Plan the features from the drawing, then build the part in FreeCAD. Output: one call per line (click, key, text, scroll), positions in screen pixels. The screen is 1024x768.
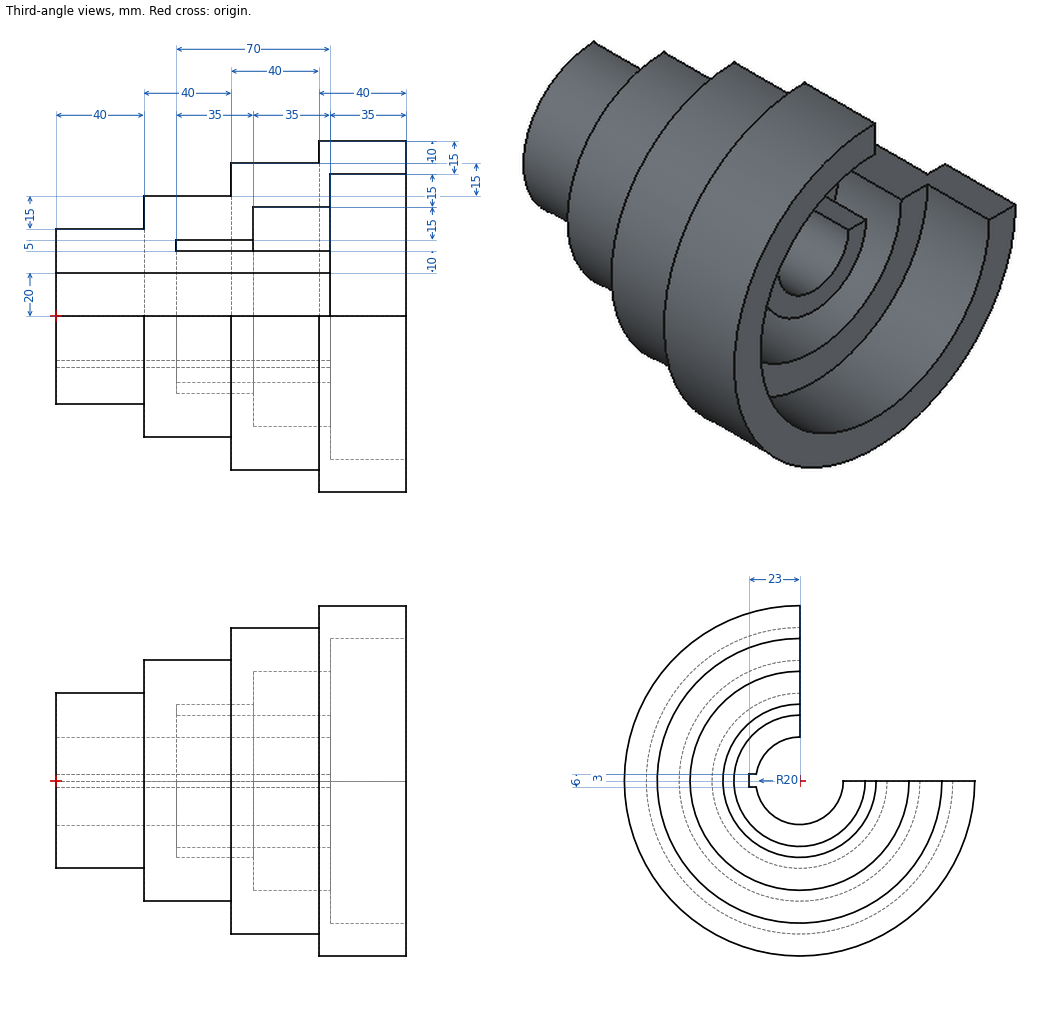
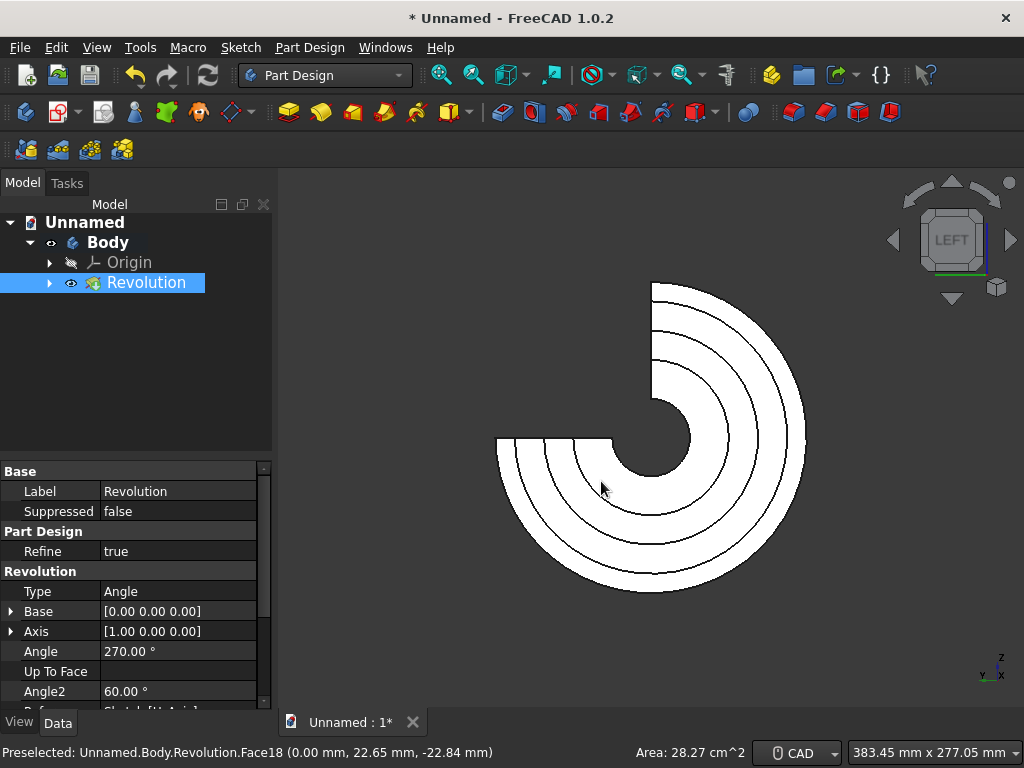
click(58, 112)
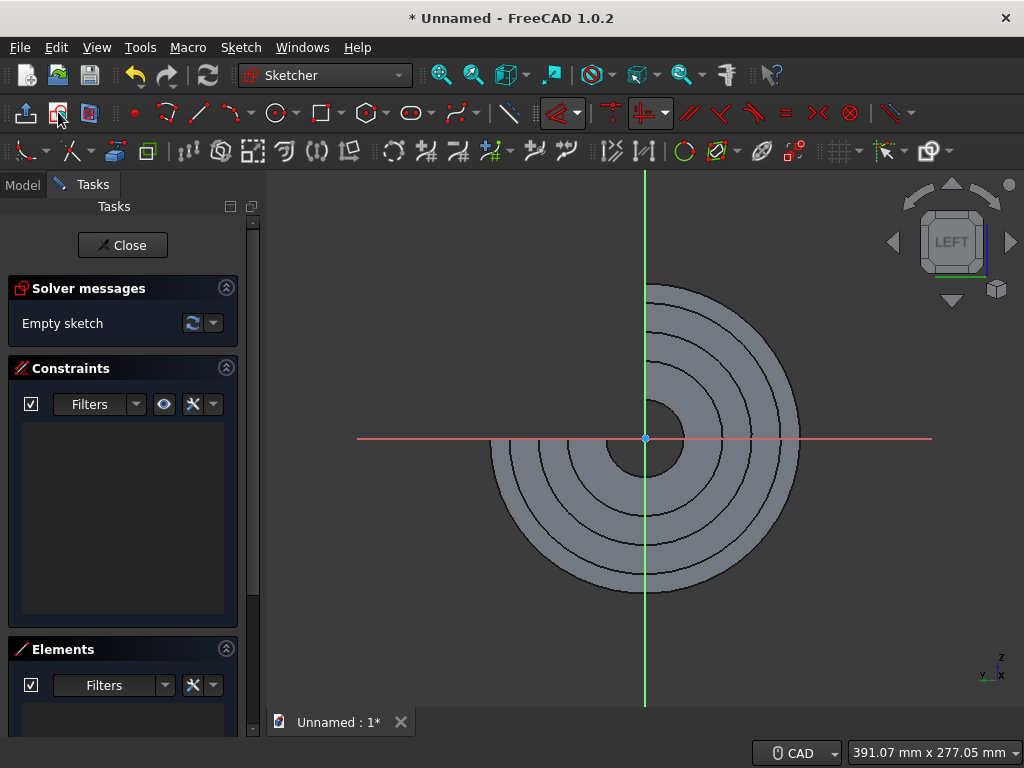
scroll(692, 439, up, 15)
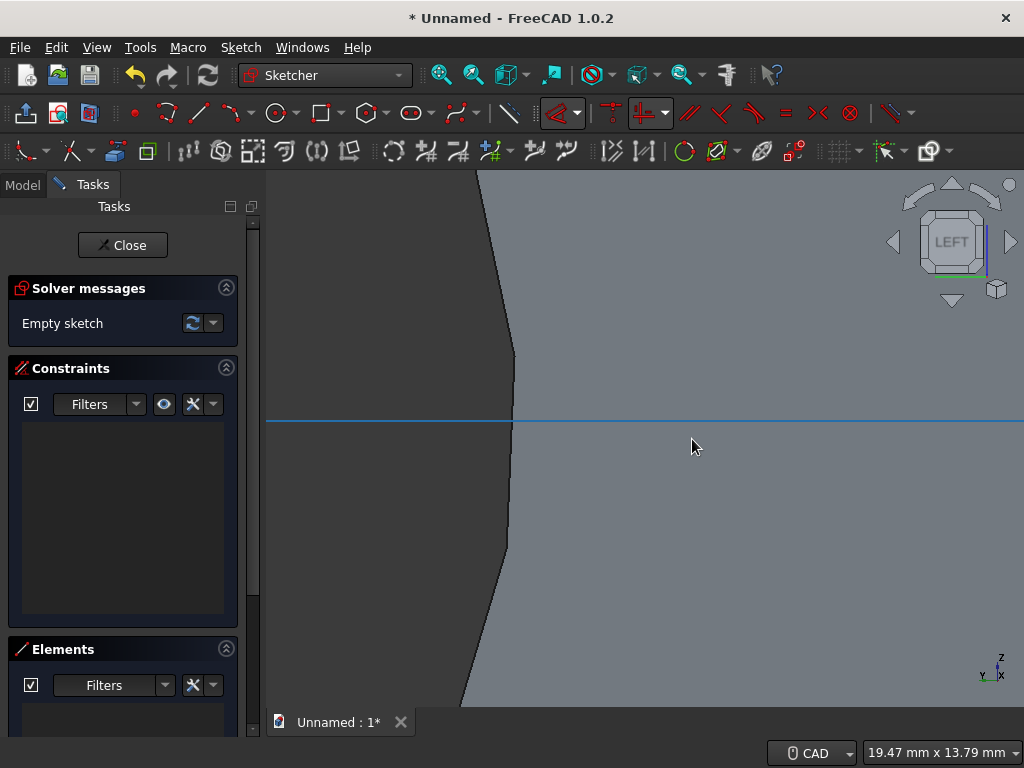
scroll(560, 385, up, 2)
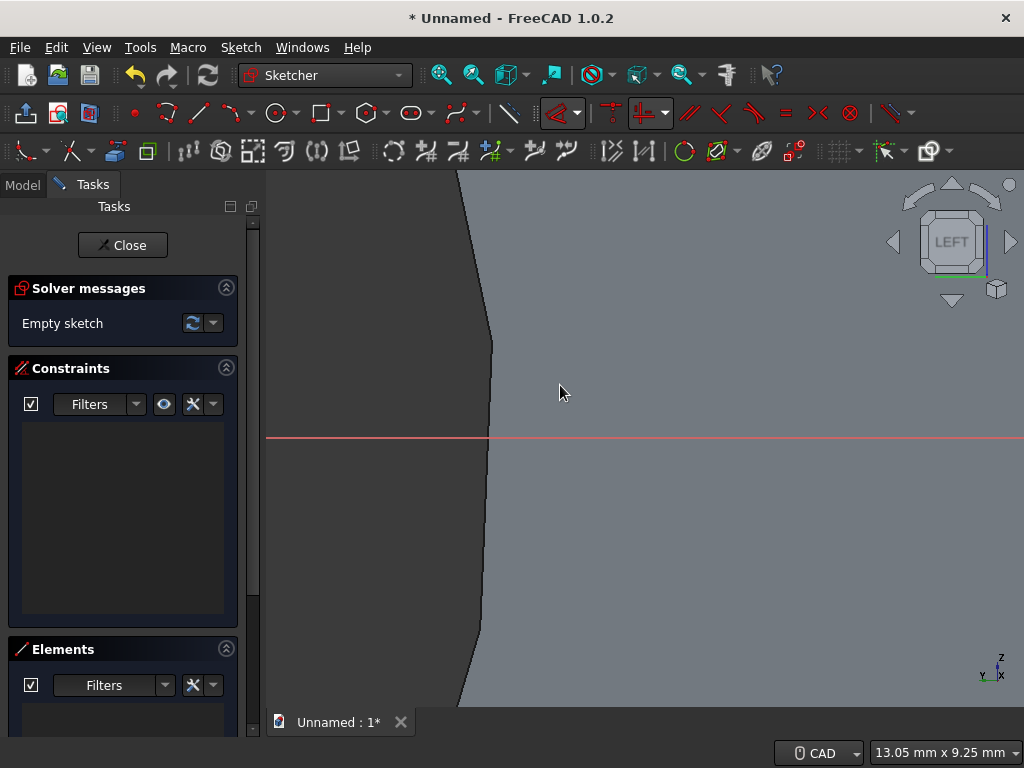
click(168, 114)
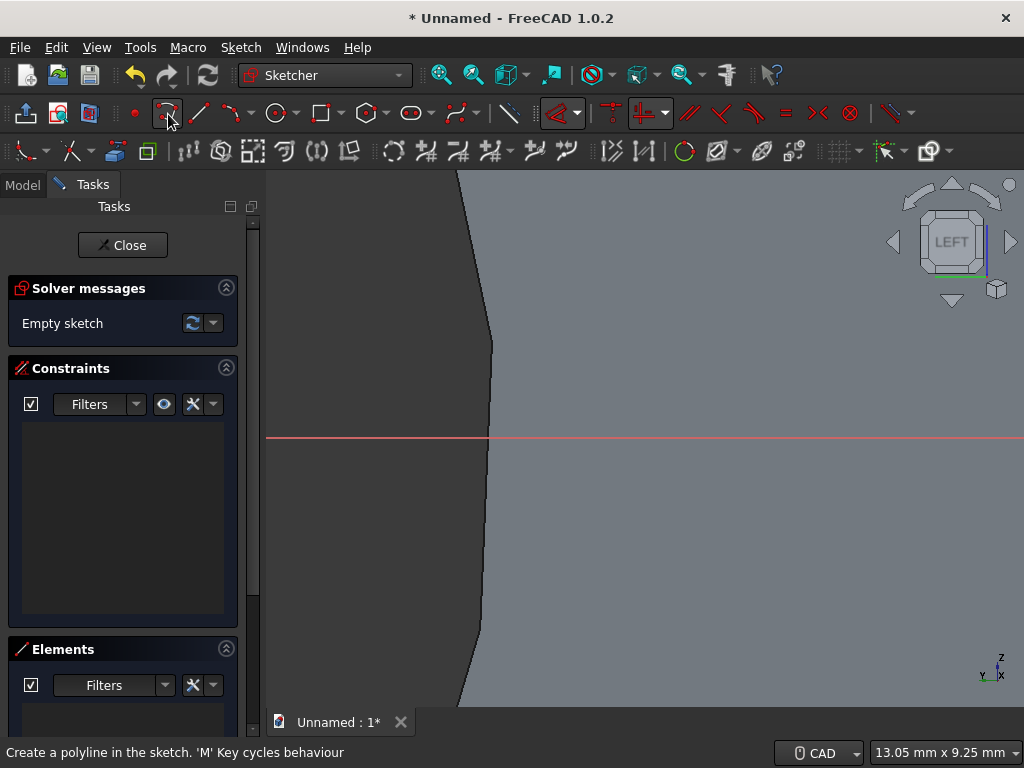
click(483, 264)
click(670, 264)
click(670, 612)
click(483, 612)
right_click(483, 612)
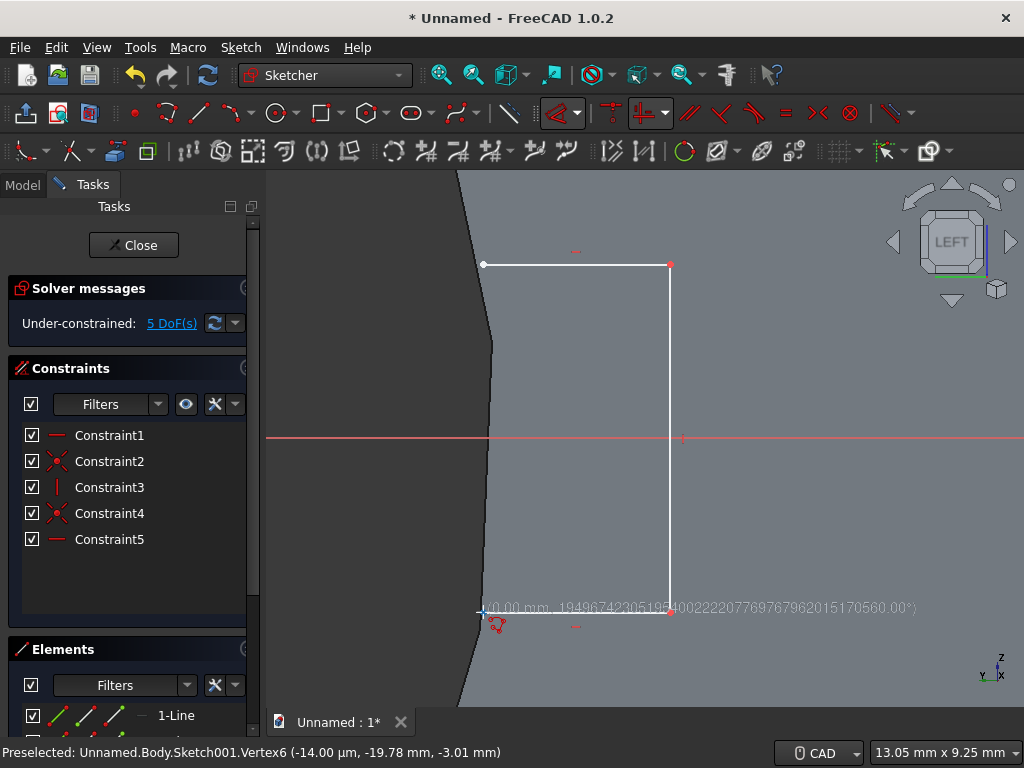
click(232, 114)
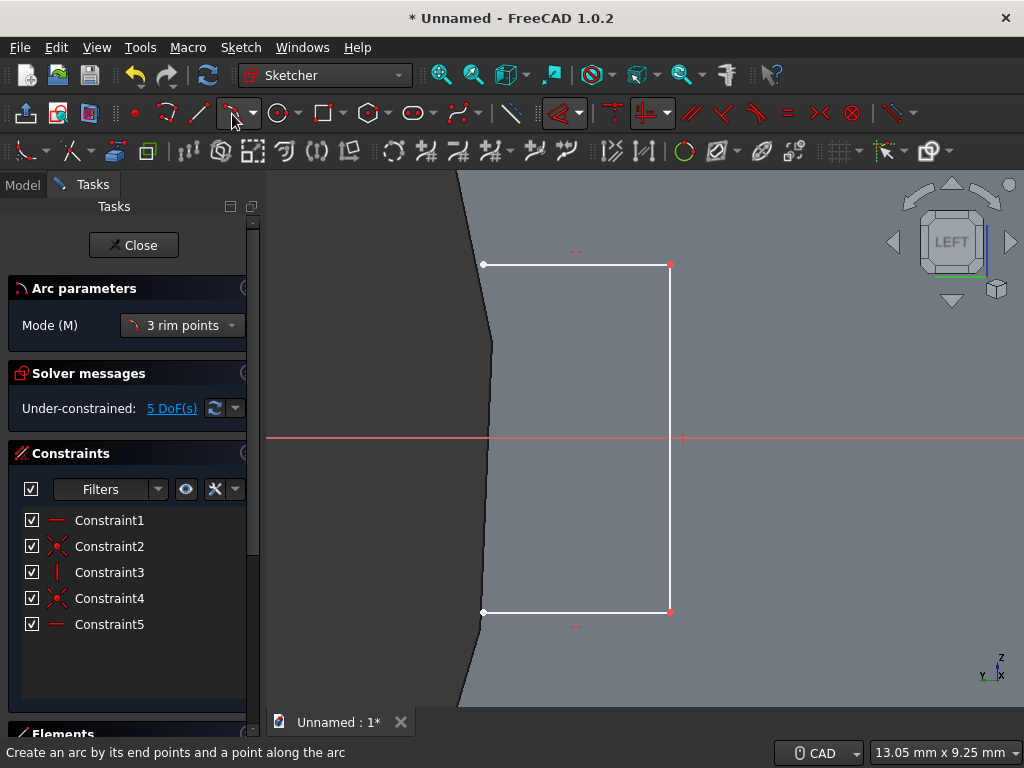
click(483, 613)
click(483, 265)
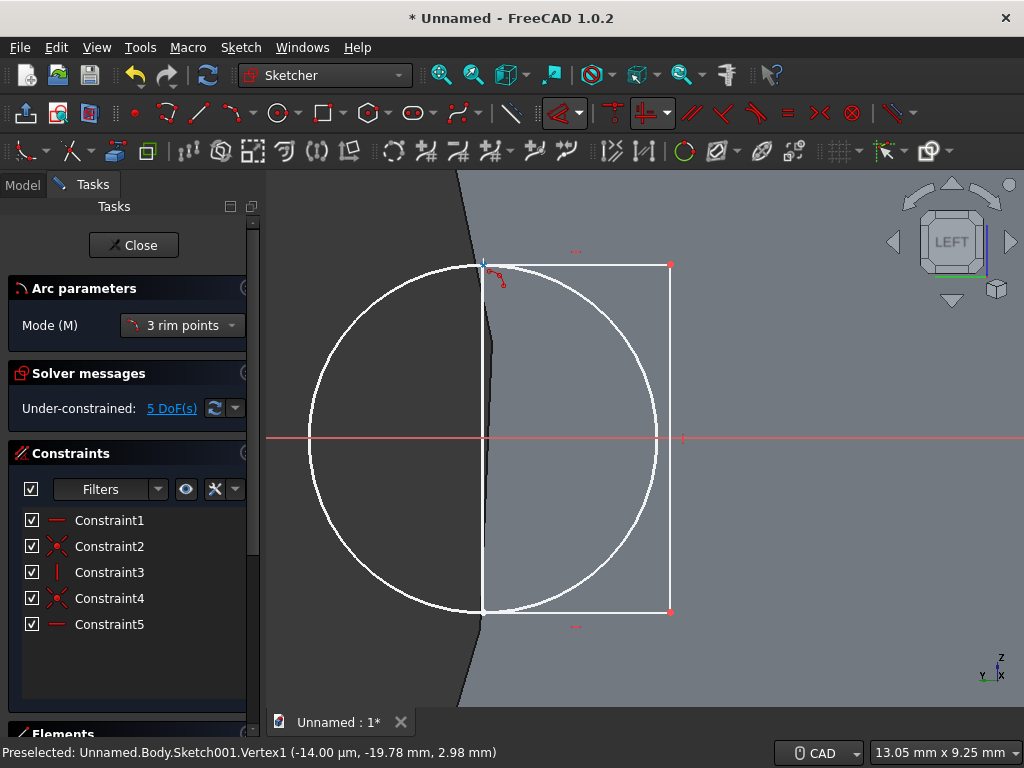
scroll(495, 473, up, 2)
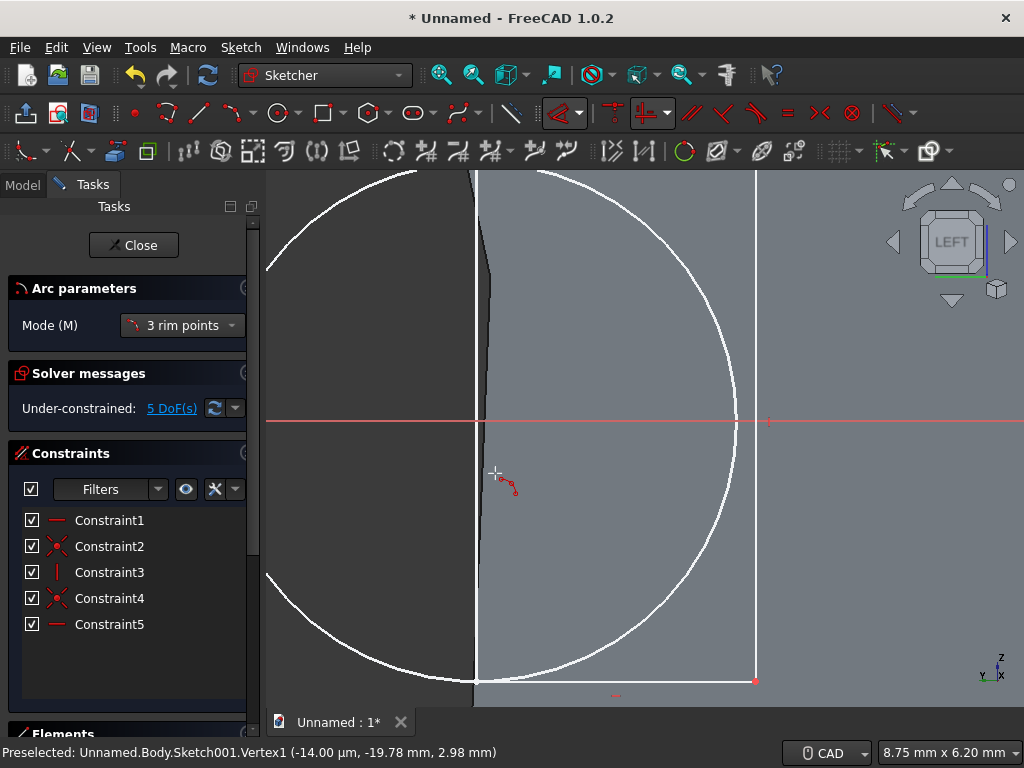
click(495, 473)
key(Escape)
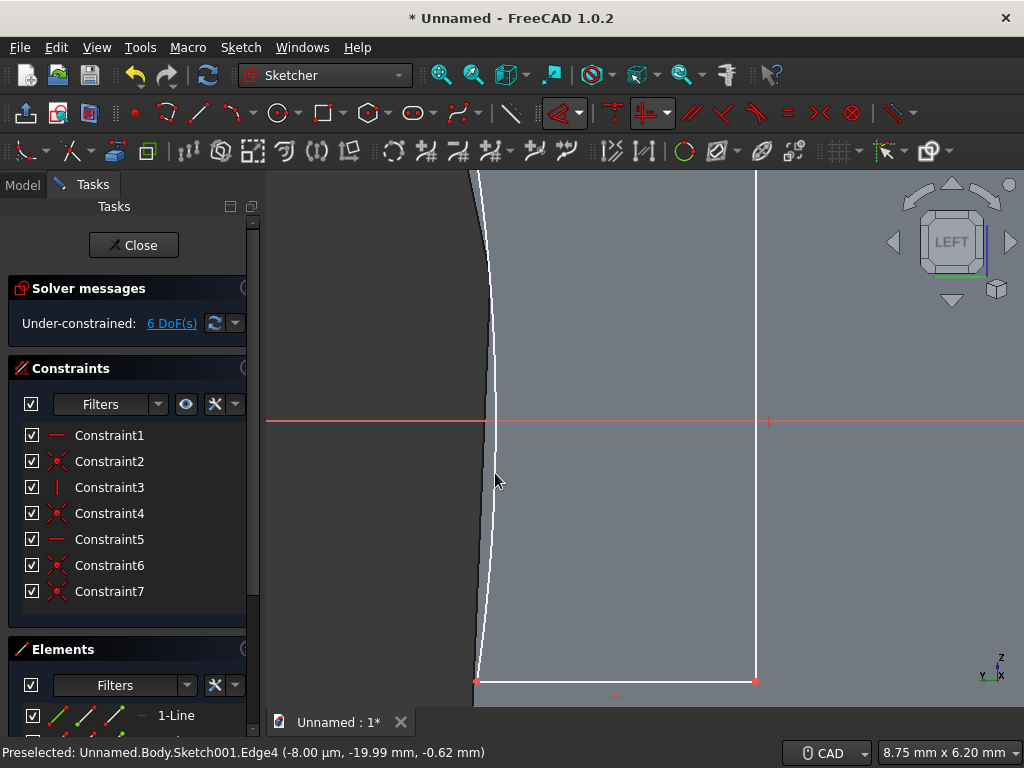
scroll(495, 475, down, 2)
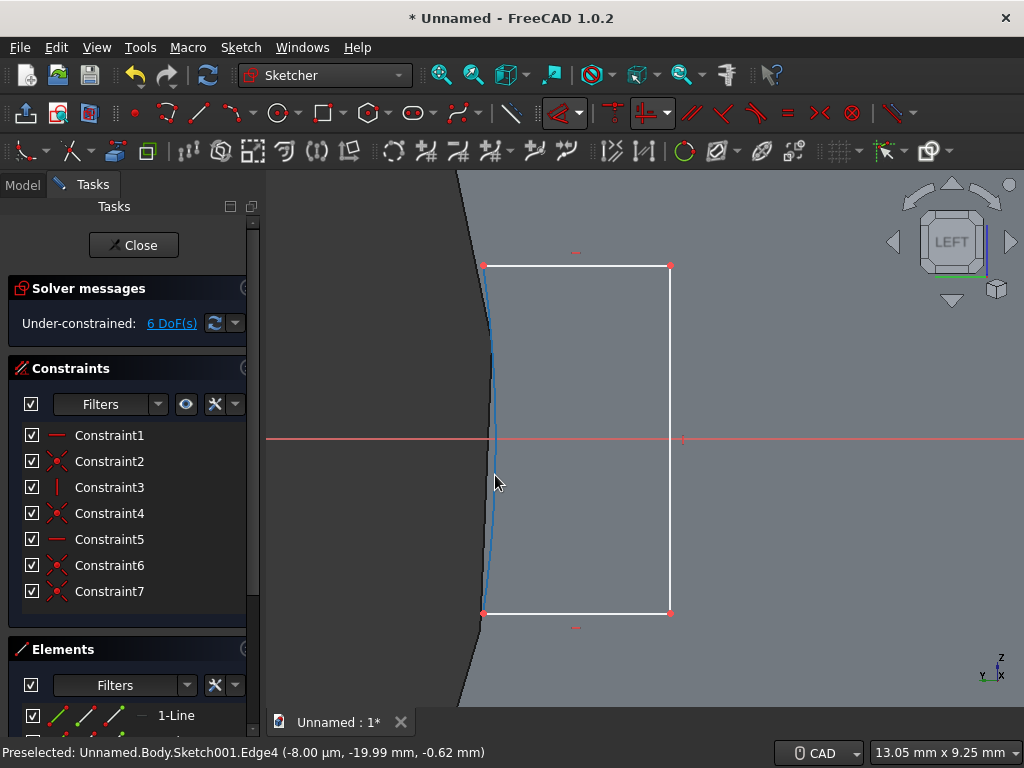
scroll(829, 438, down, 6)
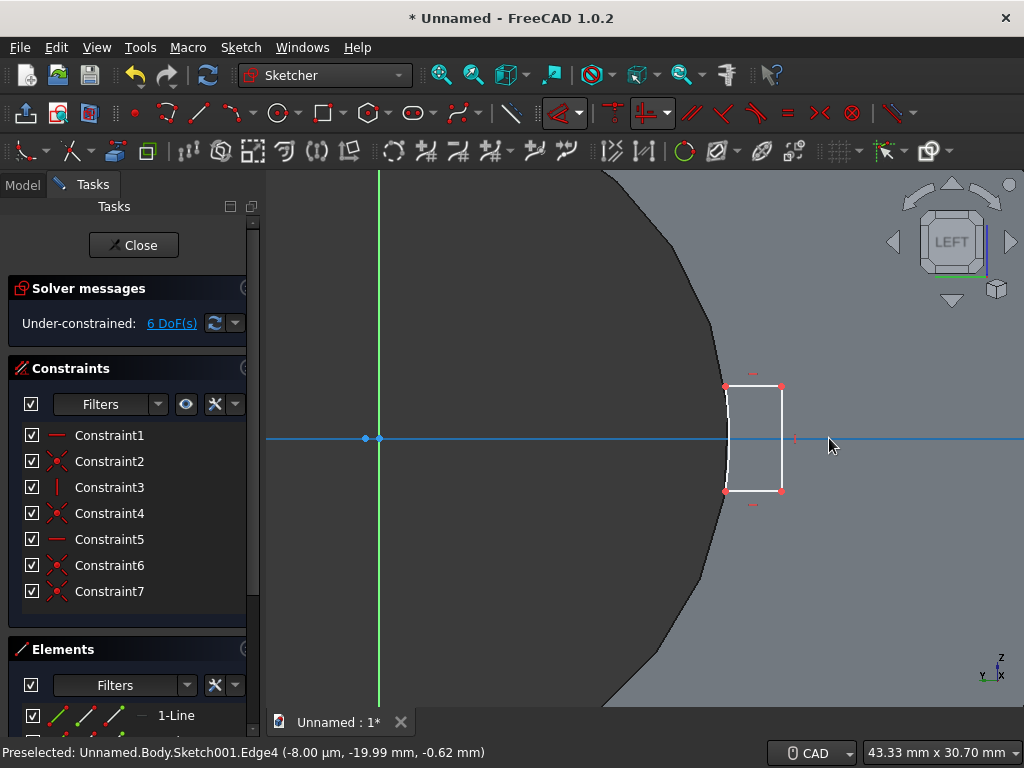
drag(355, 429, 389, 449)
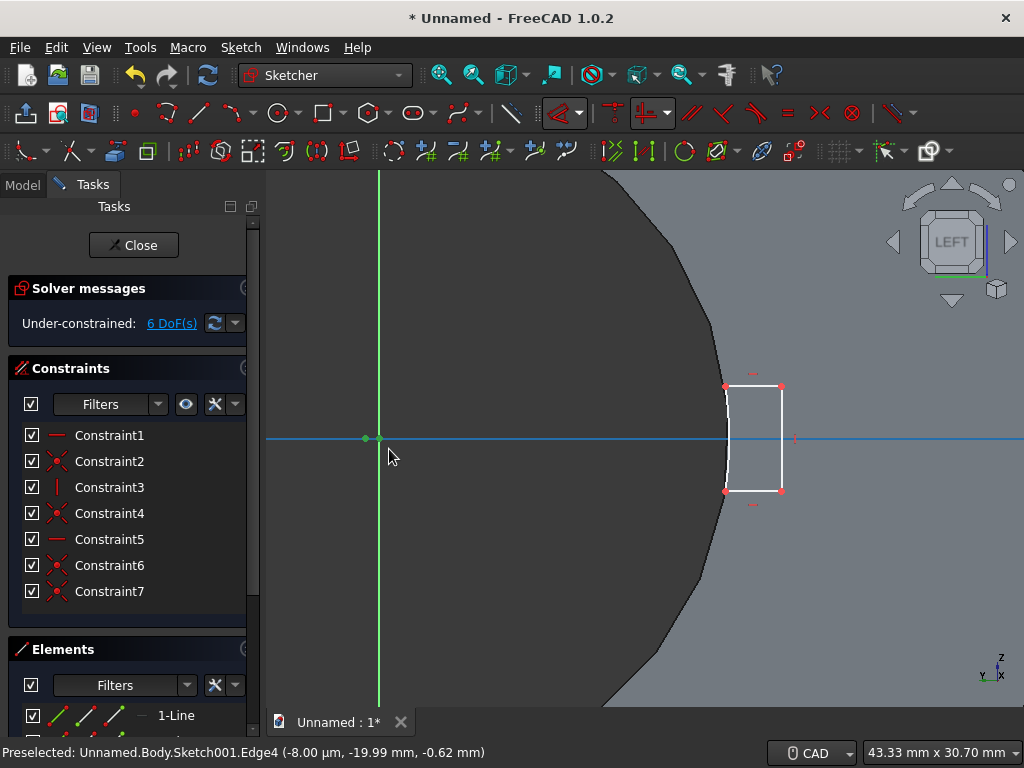
click(614, 114)